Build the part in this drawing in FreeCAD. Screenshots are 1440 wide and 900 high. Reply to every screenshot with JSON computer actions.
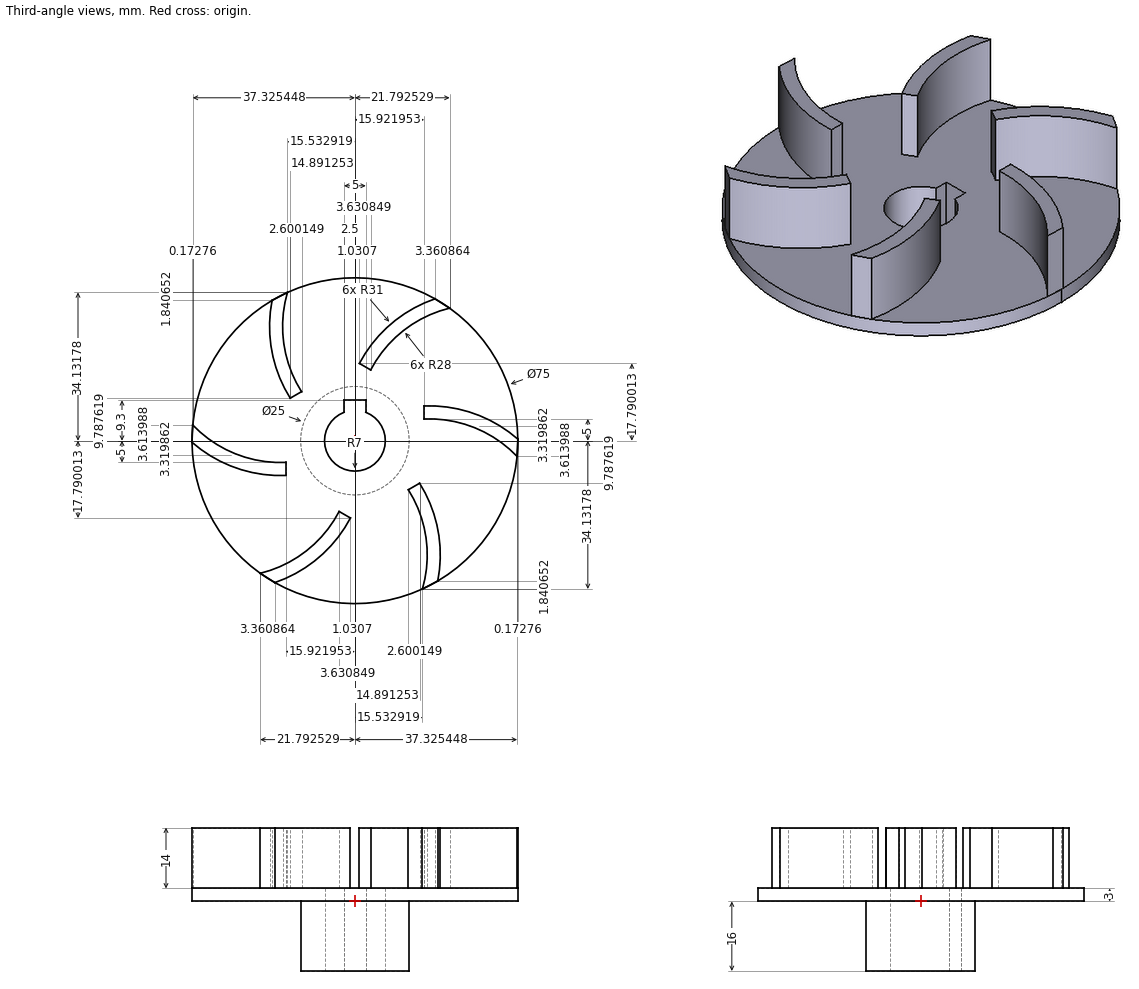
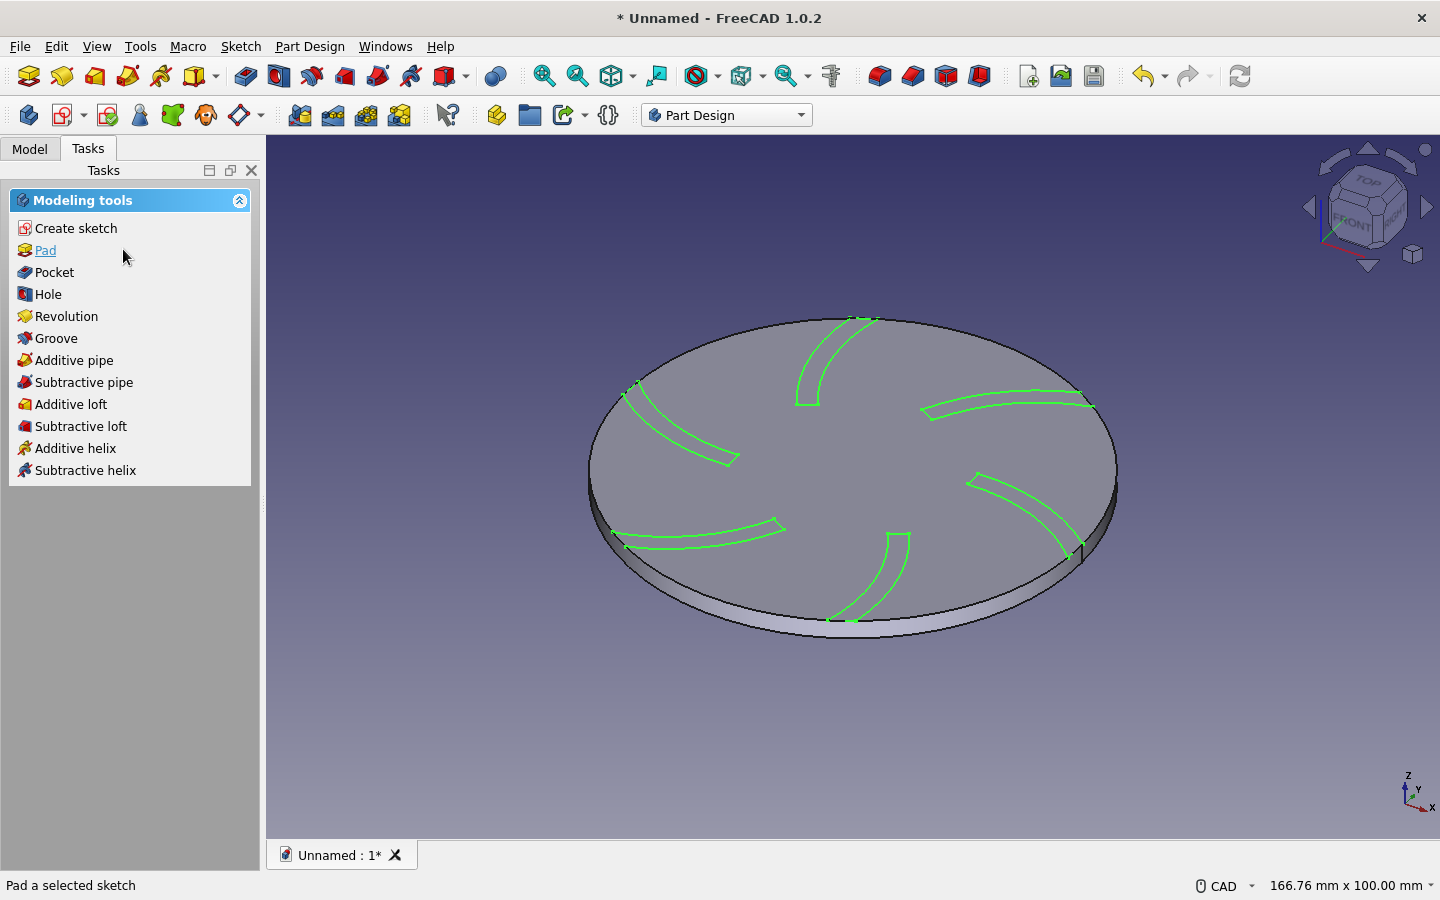
{"action": "left_click", "coordinate": [29, 76]}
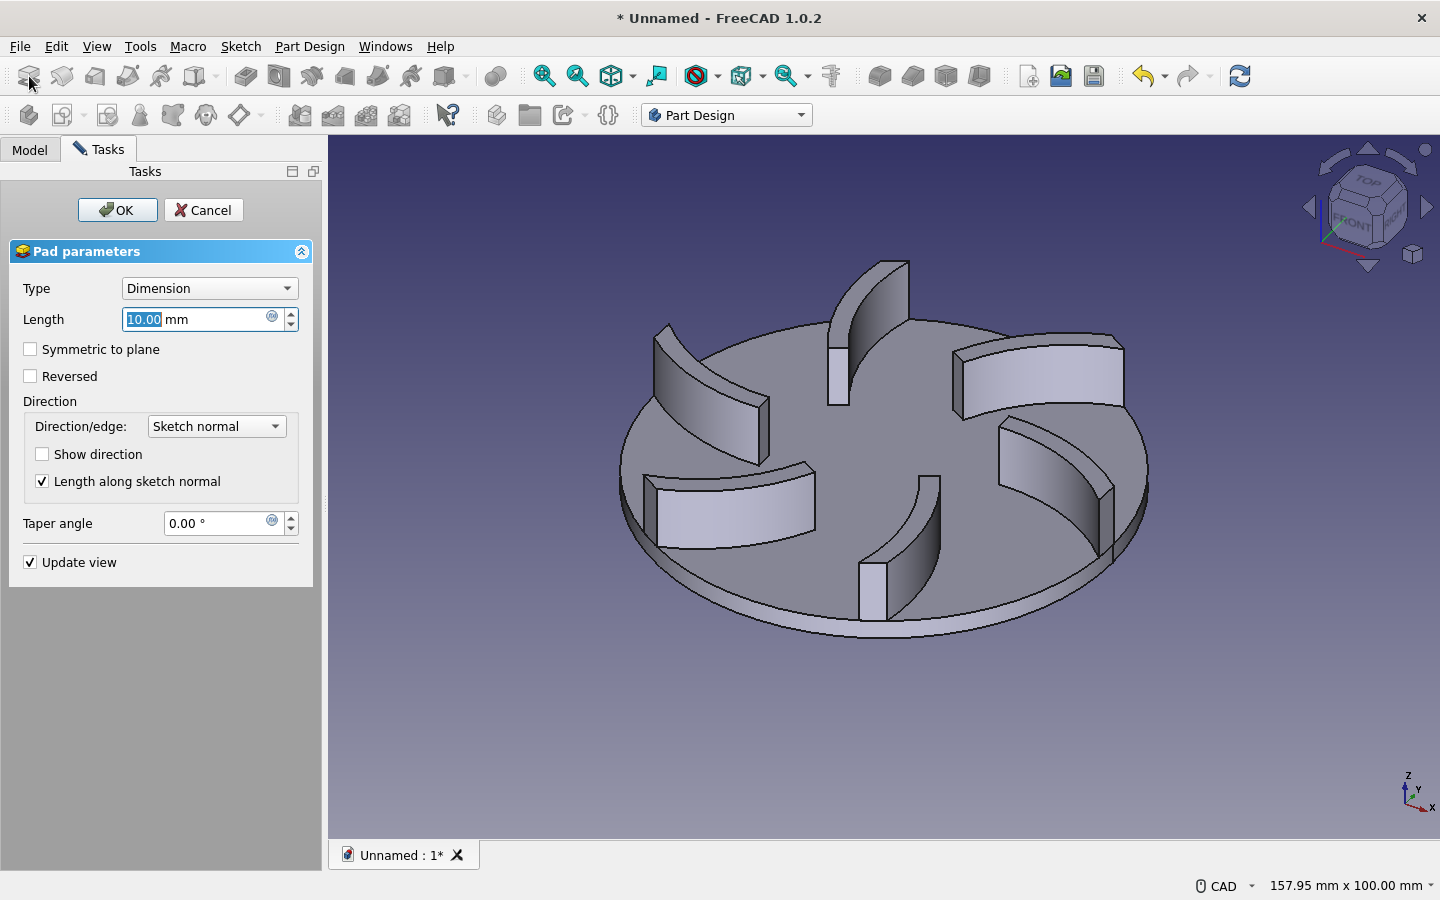
{"action": "type", "text": "14"}
{"action": "key", "text": "Tab"}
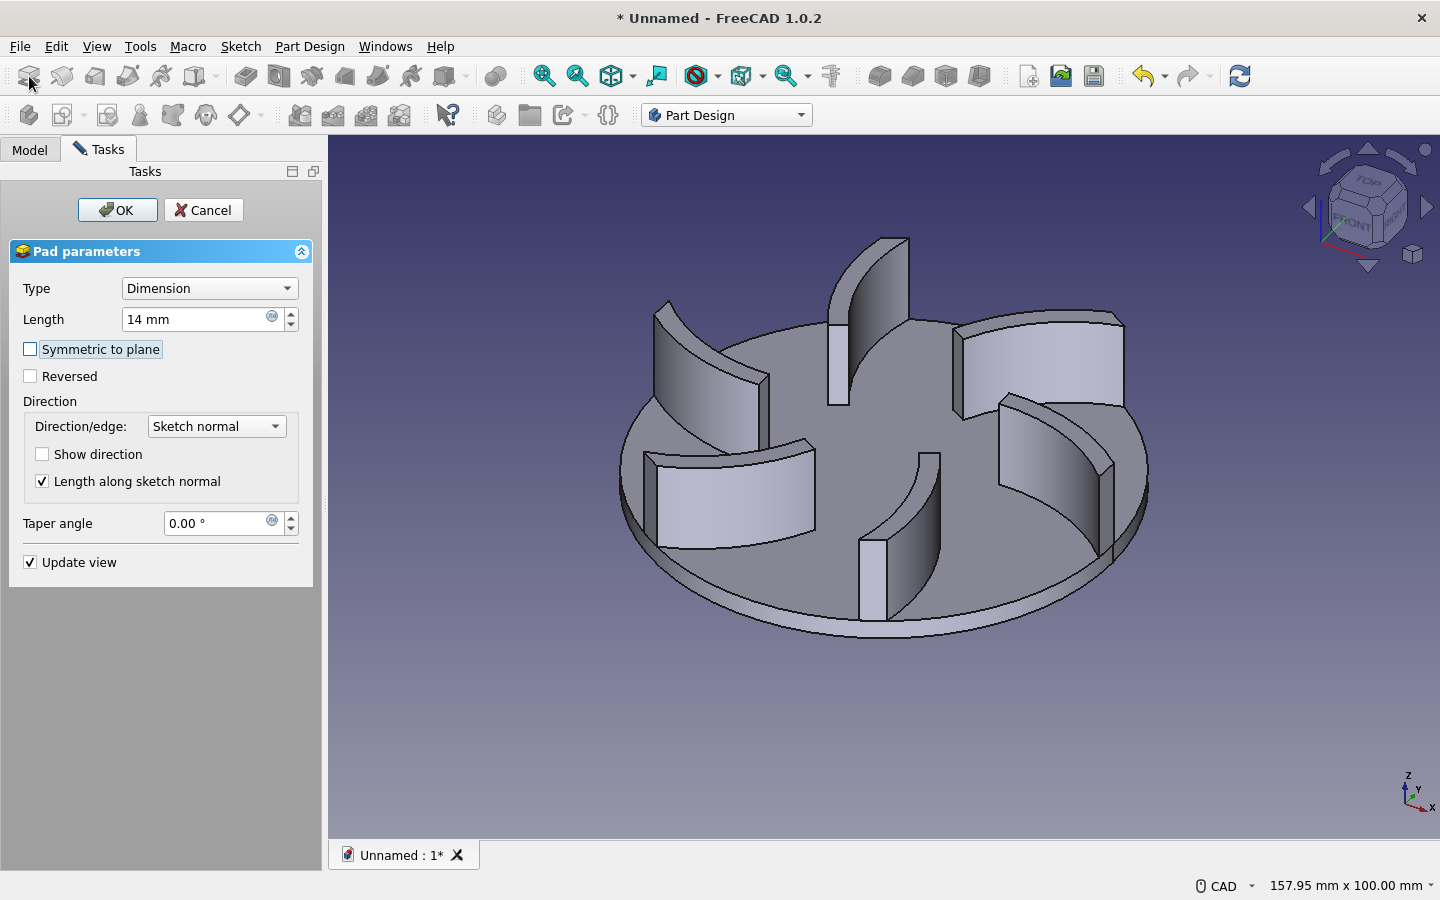
{"action": "left_click", "coordinate": [118, 210]}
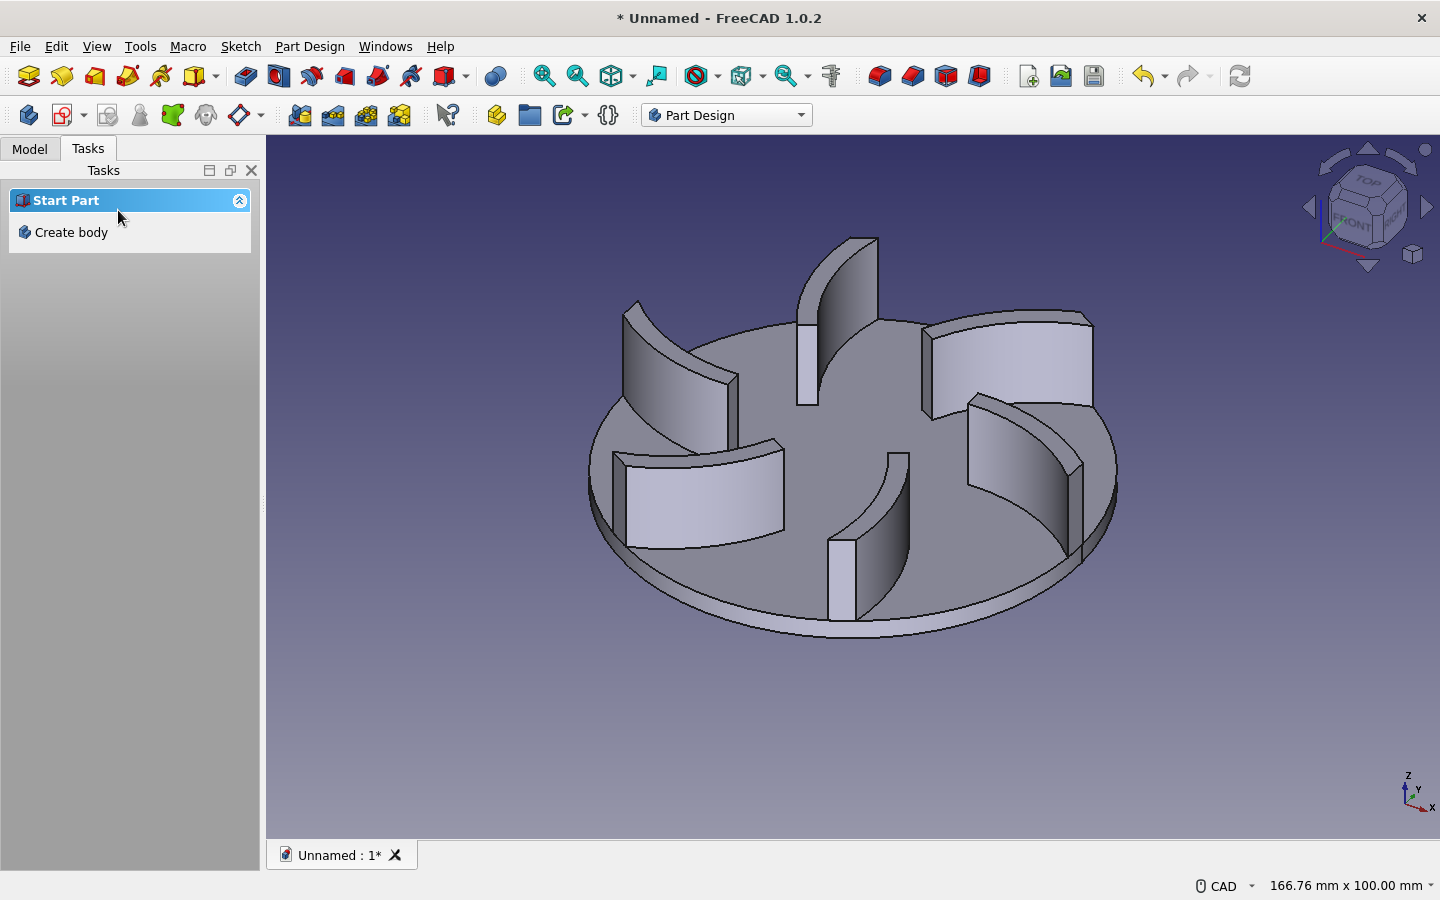
{"action": "key", "text": "5"}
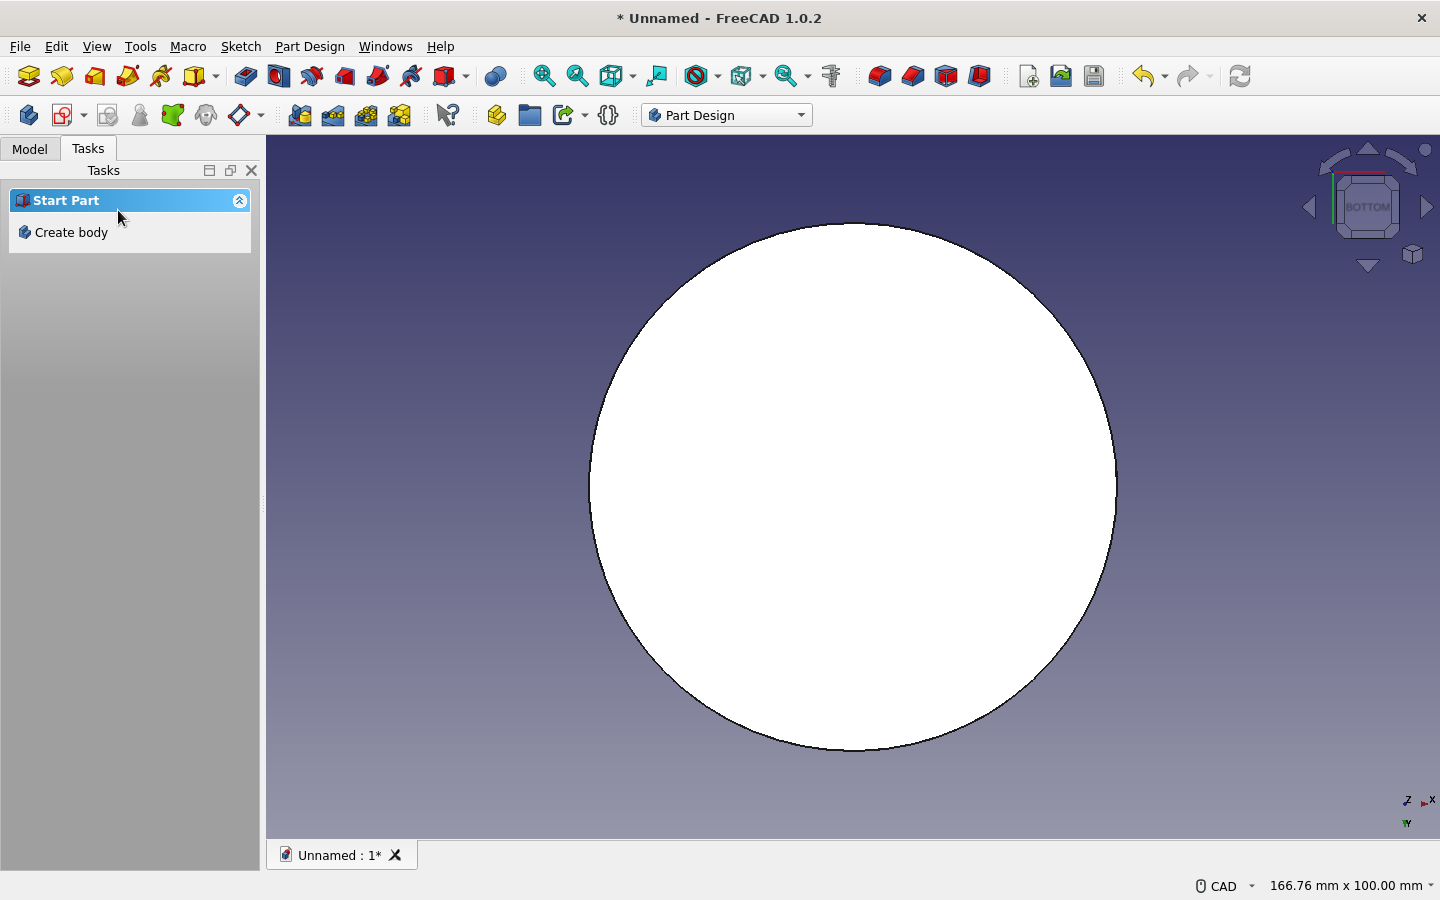
{"action": "left_click", "coordinate": [853, 486]}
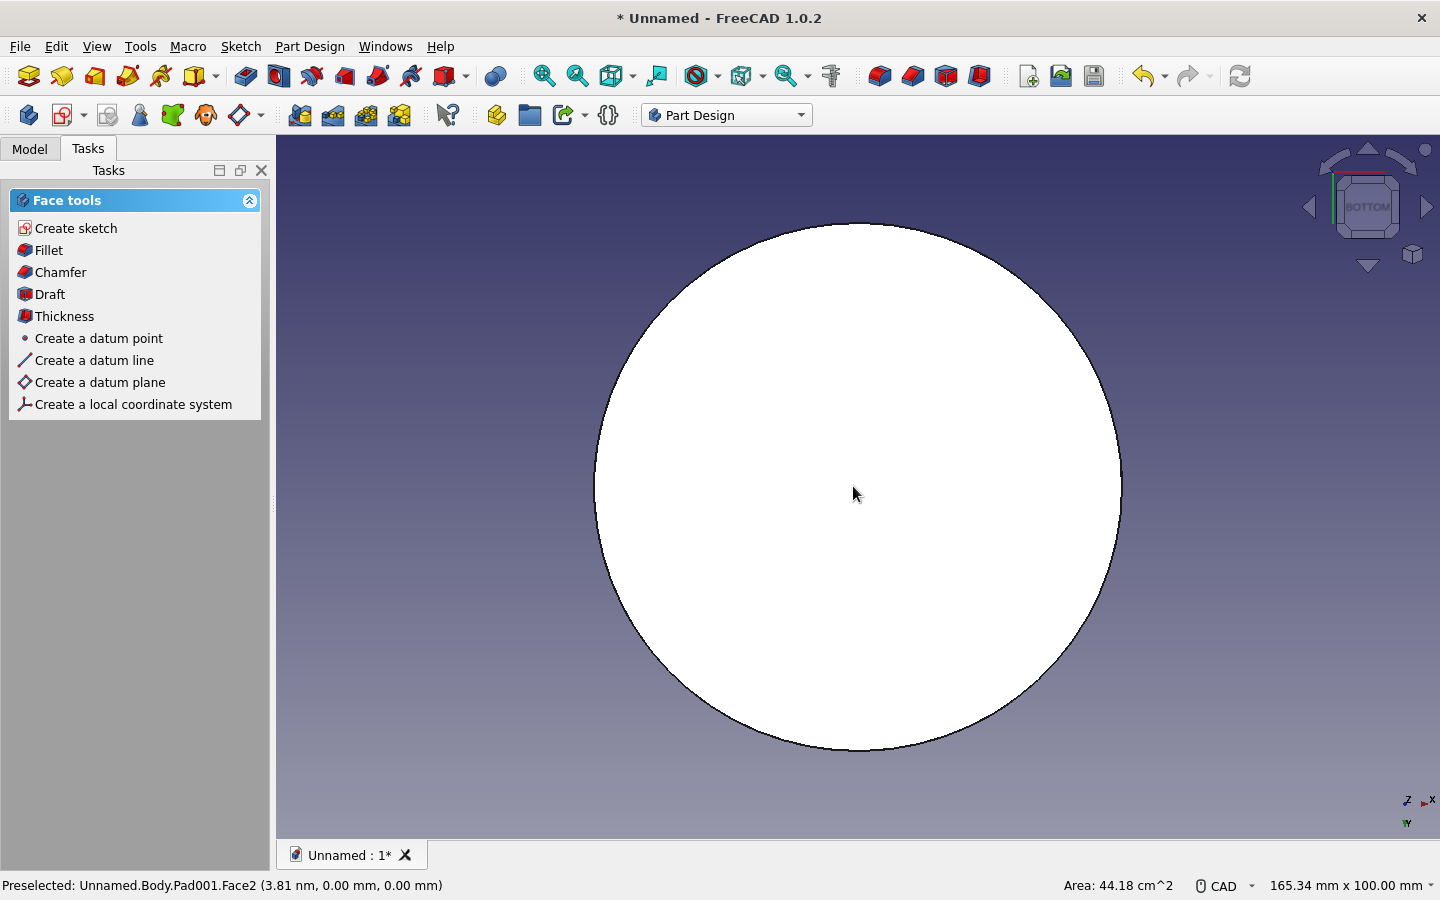
{"action": "left_click", "coordinate": [62, 116]}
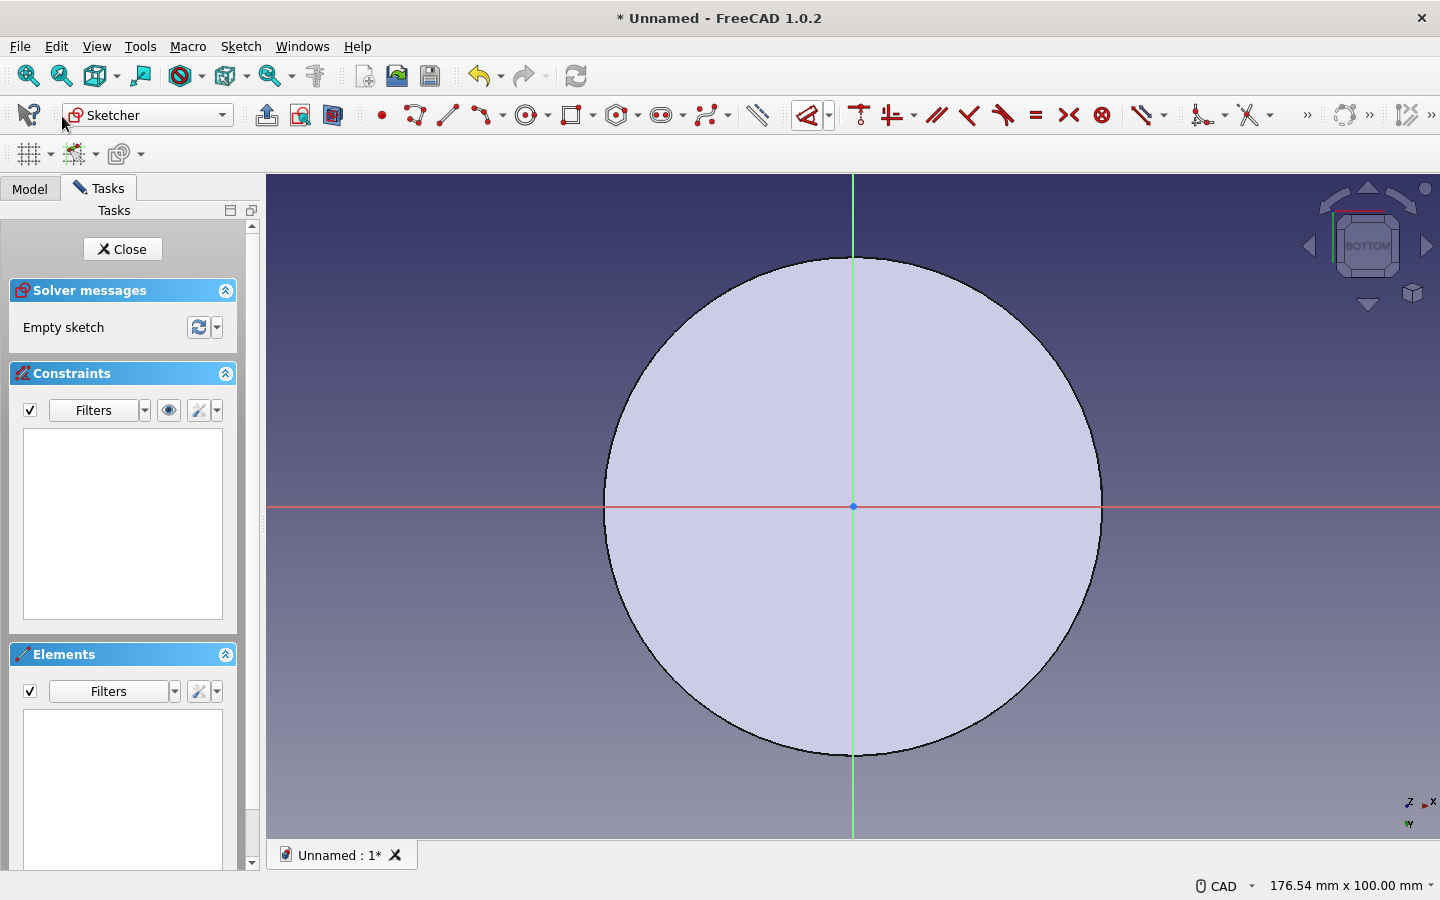
{"action": "scroll", "coordinate": [893, 507], "scroll_direction": "up", "scroll_amount": 5}